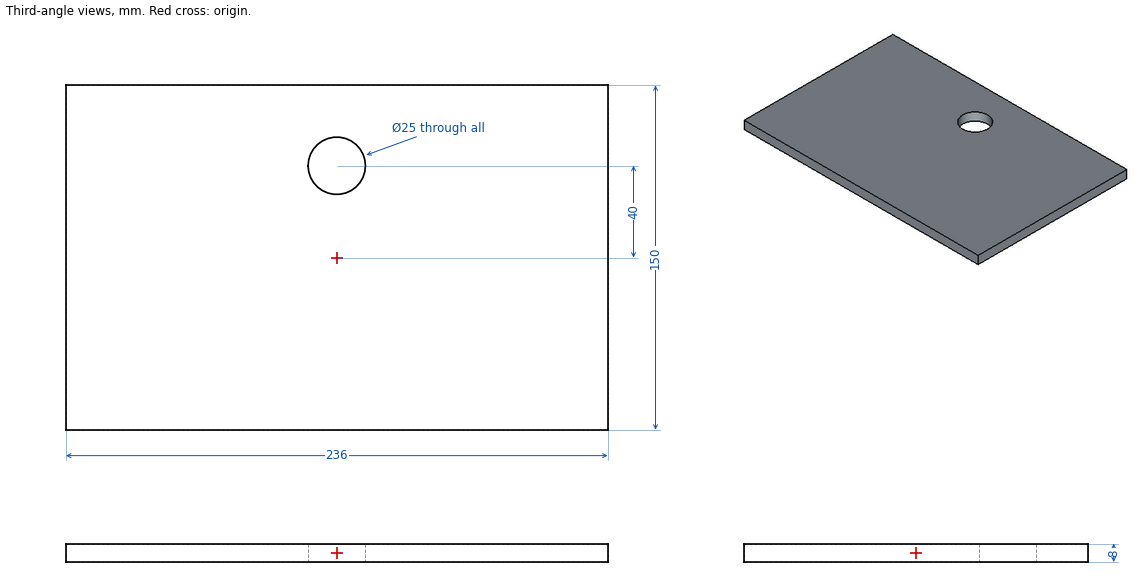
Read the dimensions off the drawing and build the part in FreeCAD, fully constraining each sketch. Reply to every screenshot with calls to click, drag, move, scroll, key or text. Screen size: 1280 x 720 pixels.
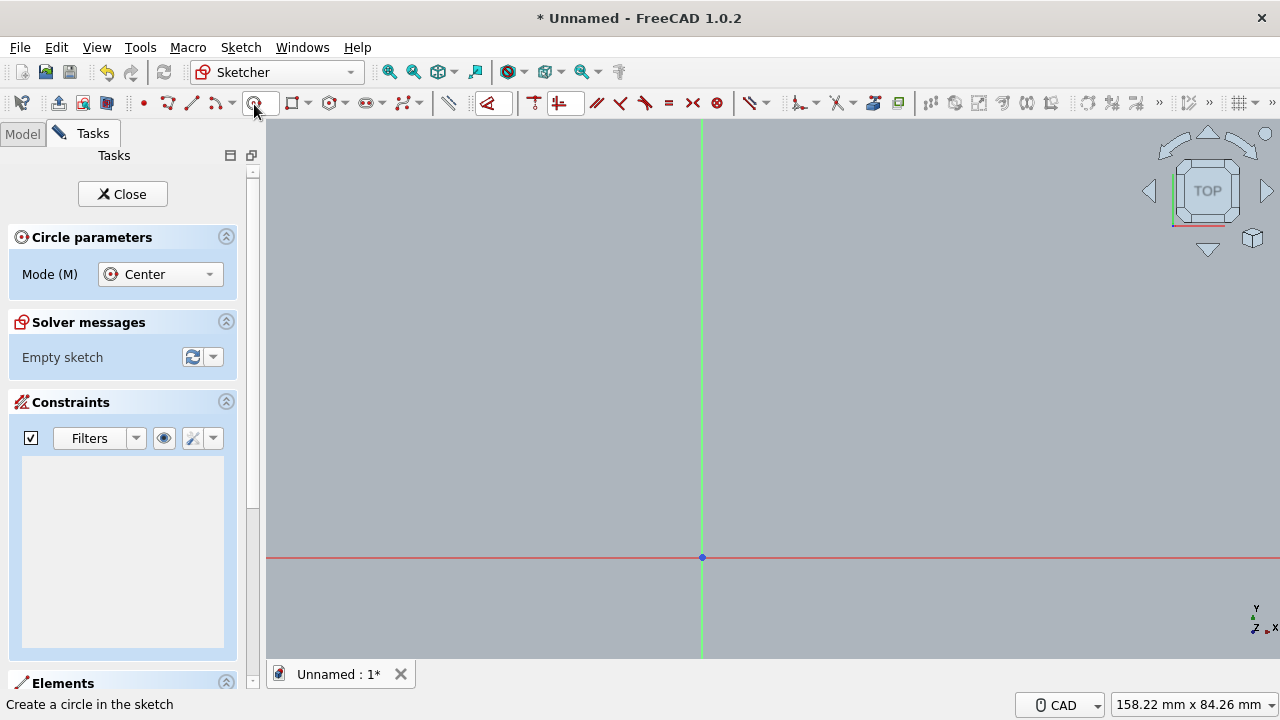
click(702, 301)
click(759, 245)
key(Escape)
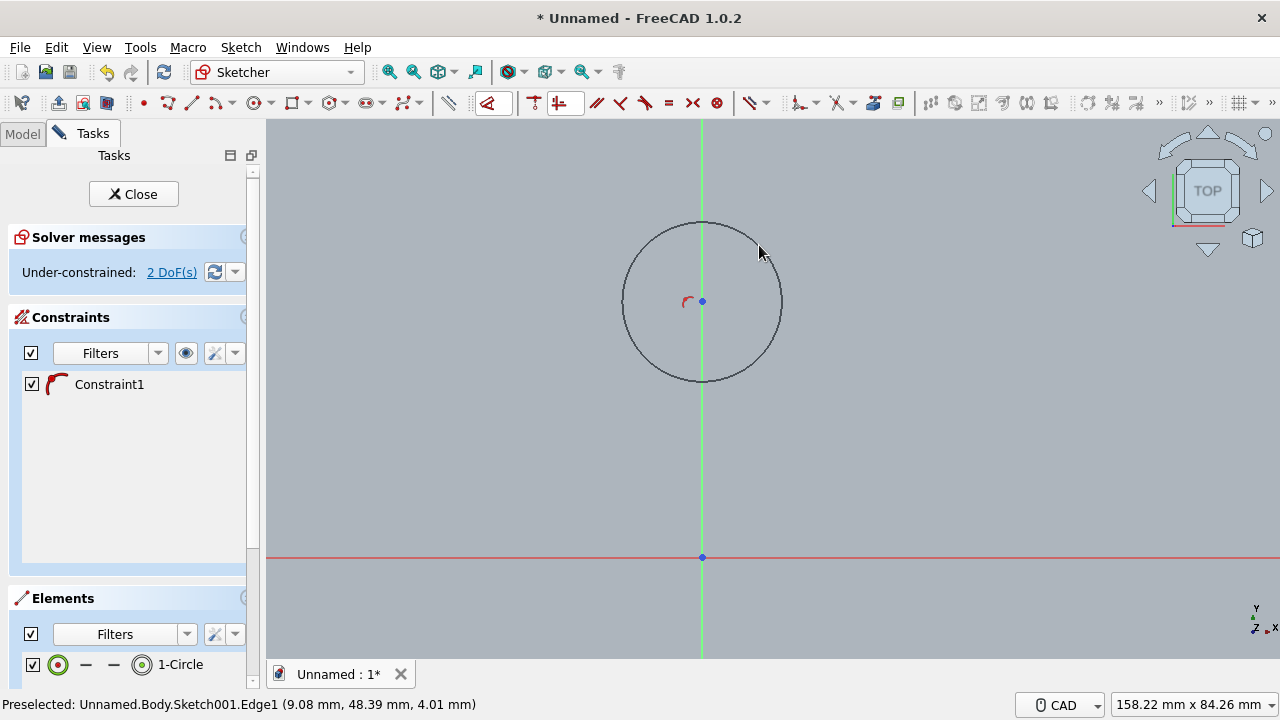
click(488, 104)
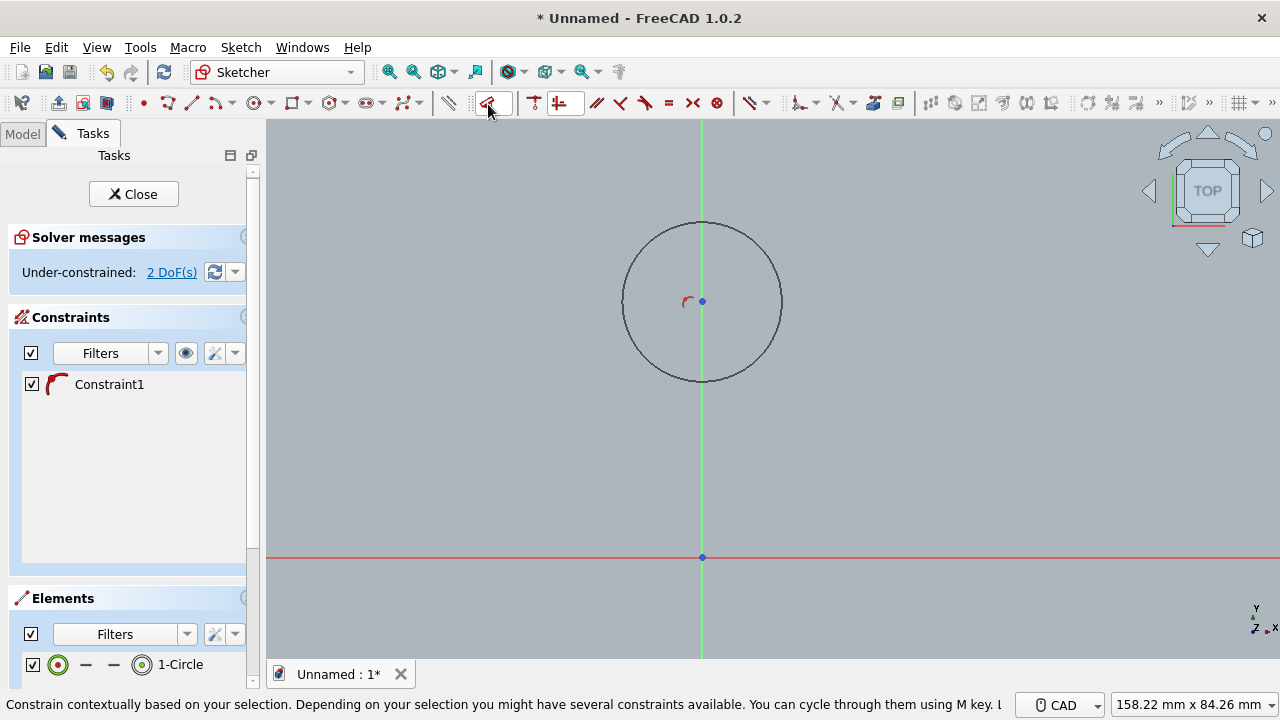
click(758, 245)
click(780, 222)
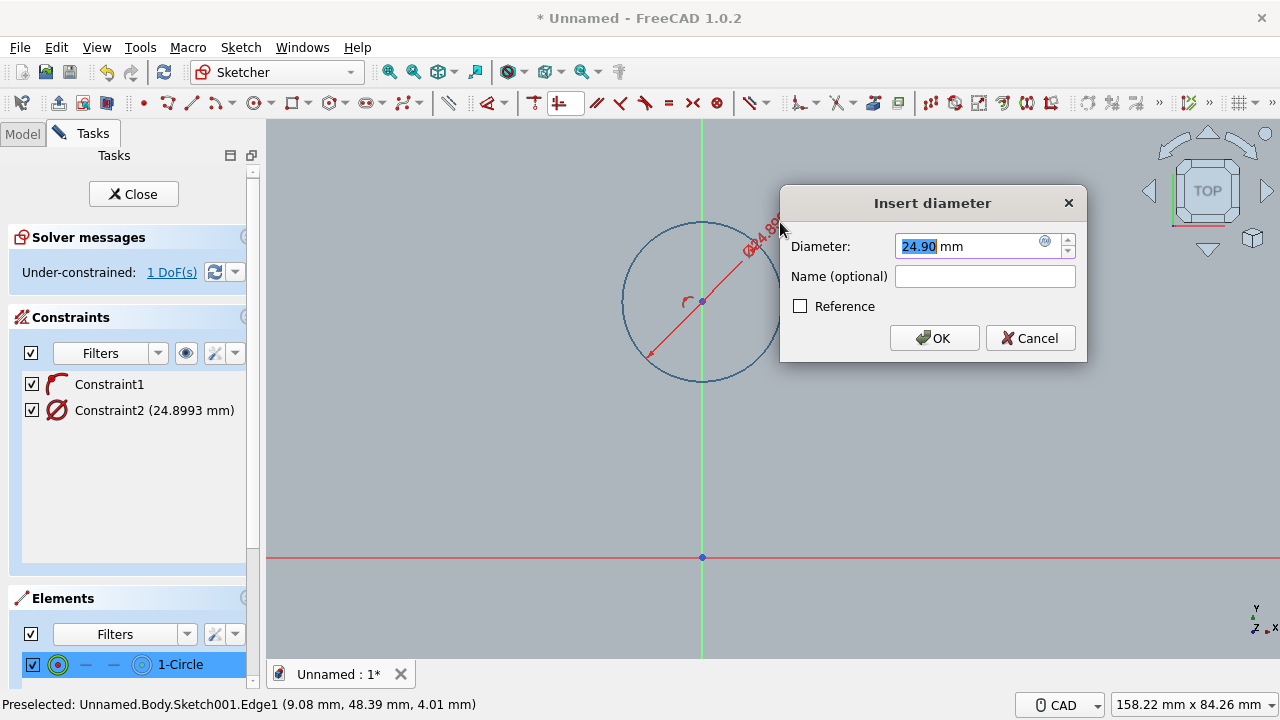
text(25)
key(Return)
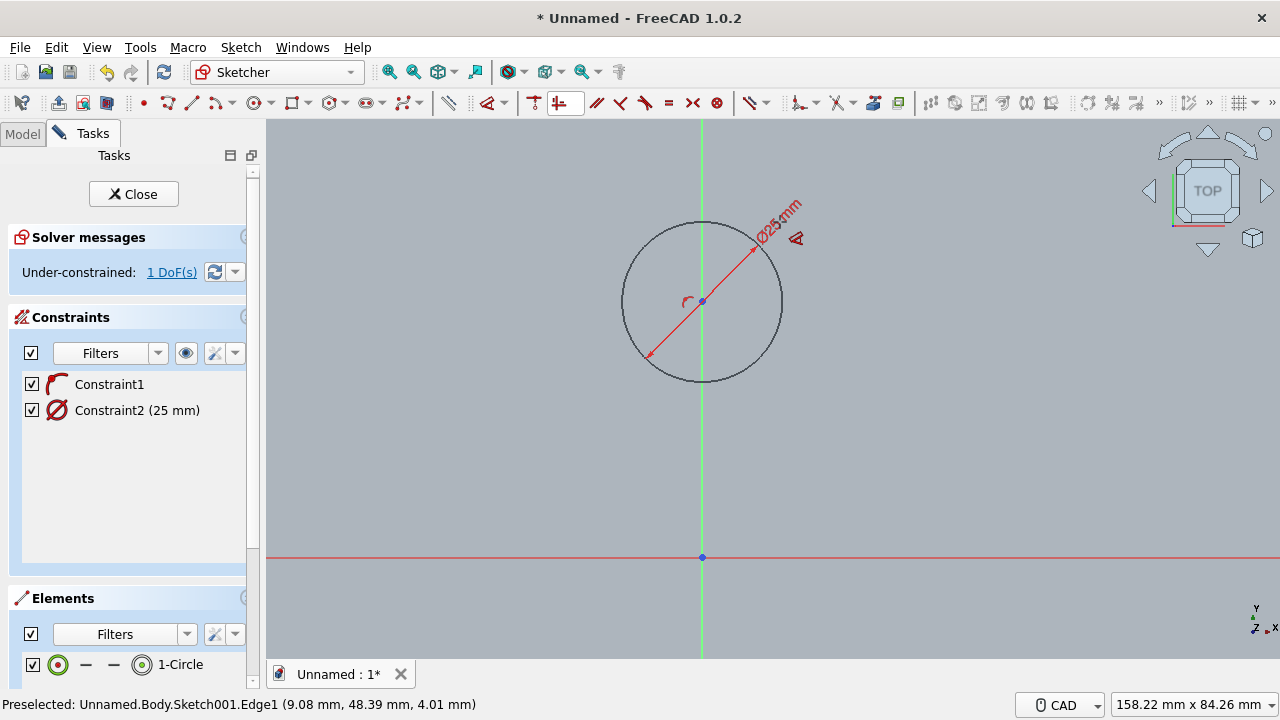
click(702, 302)
click(736, 430)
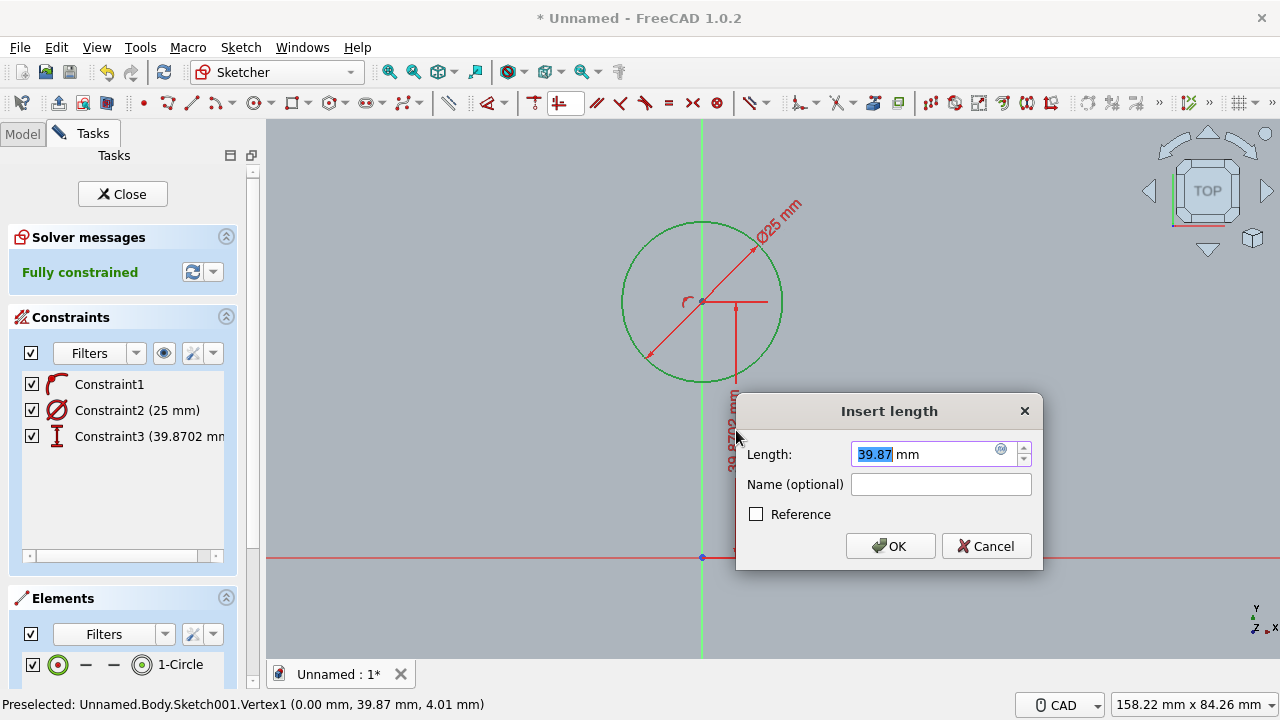
text(40)
key(Return)
key(Escape)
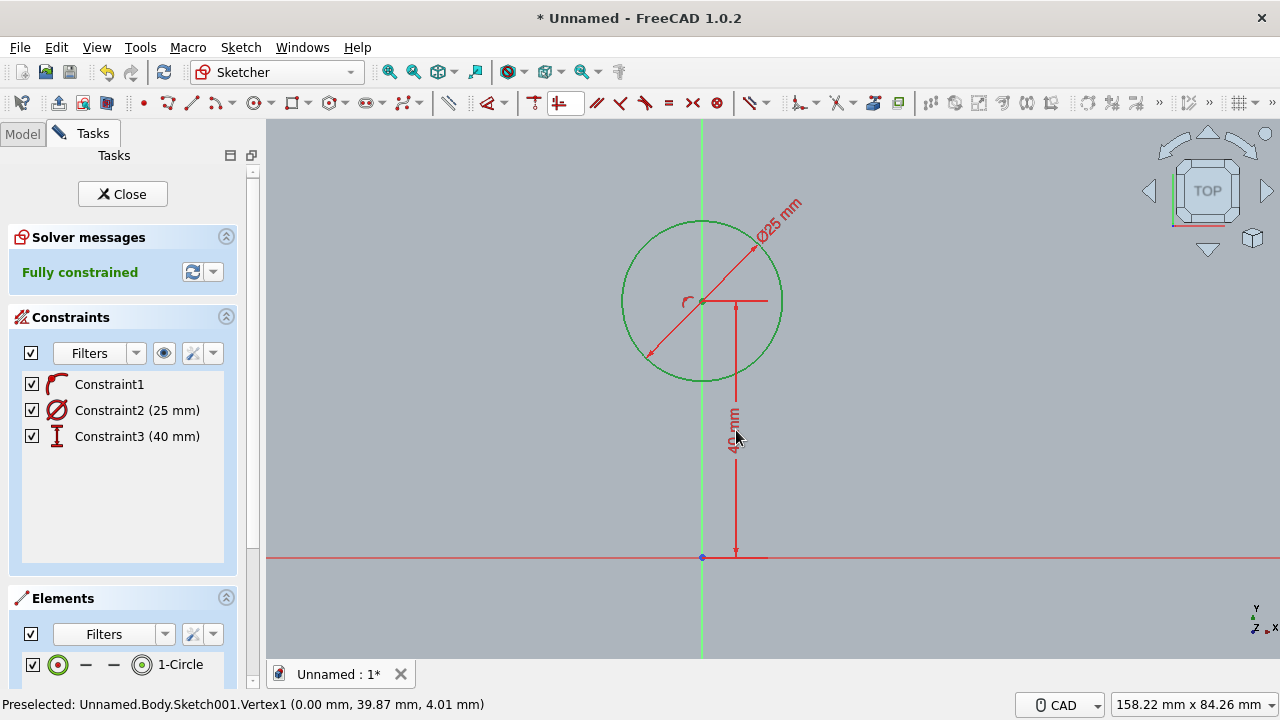
click(123, 194)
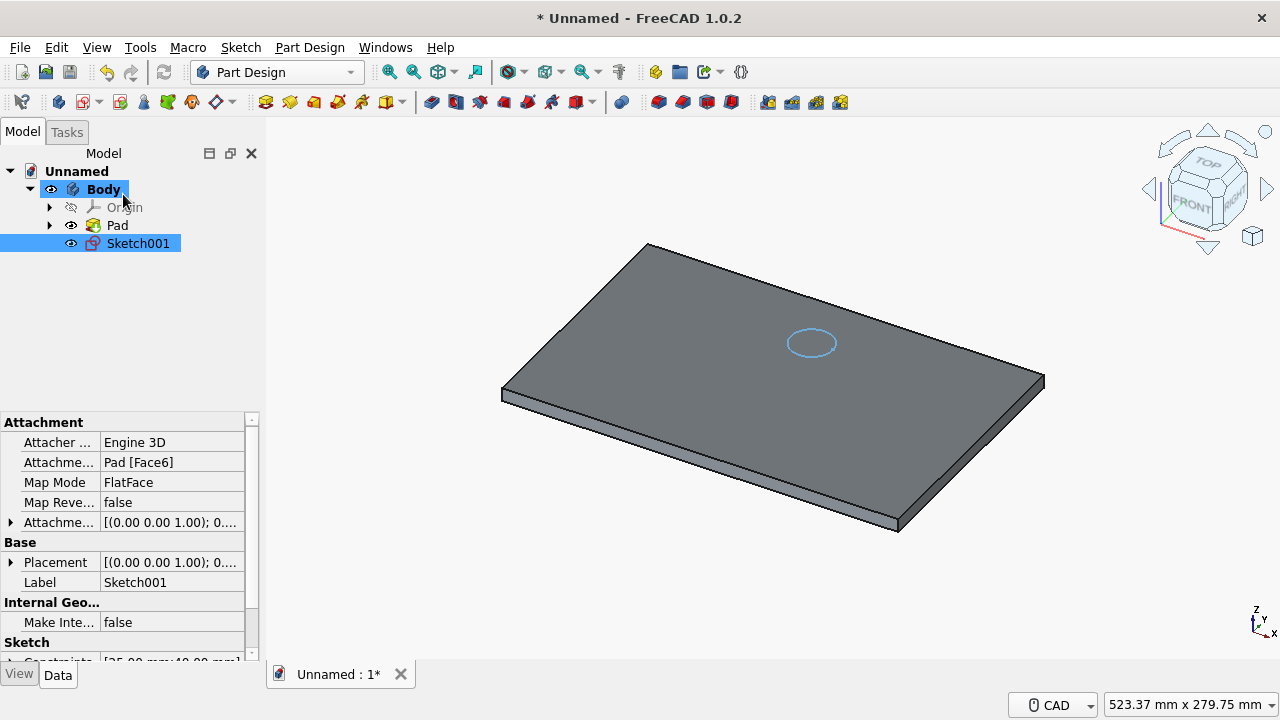
click(456, 102)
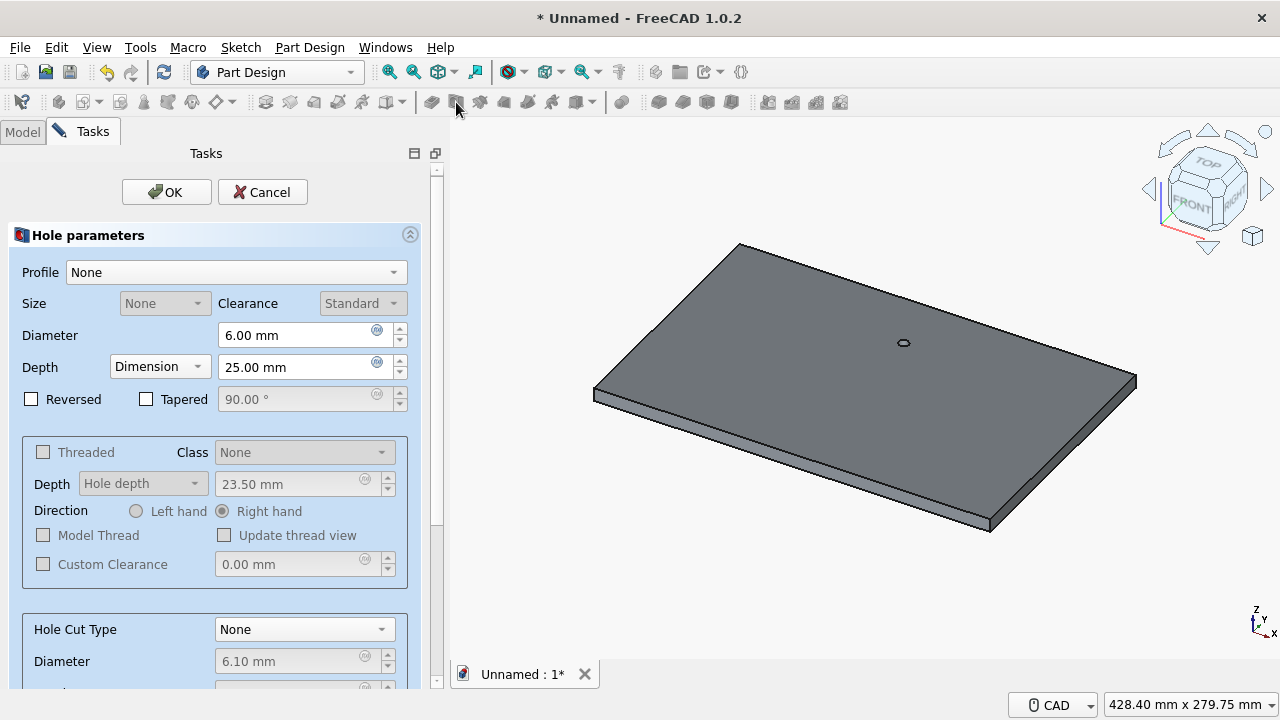
triple_click(305, 335)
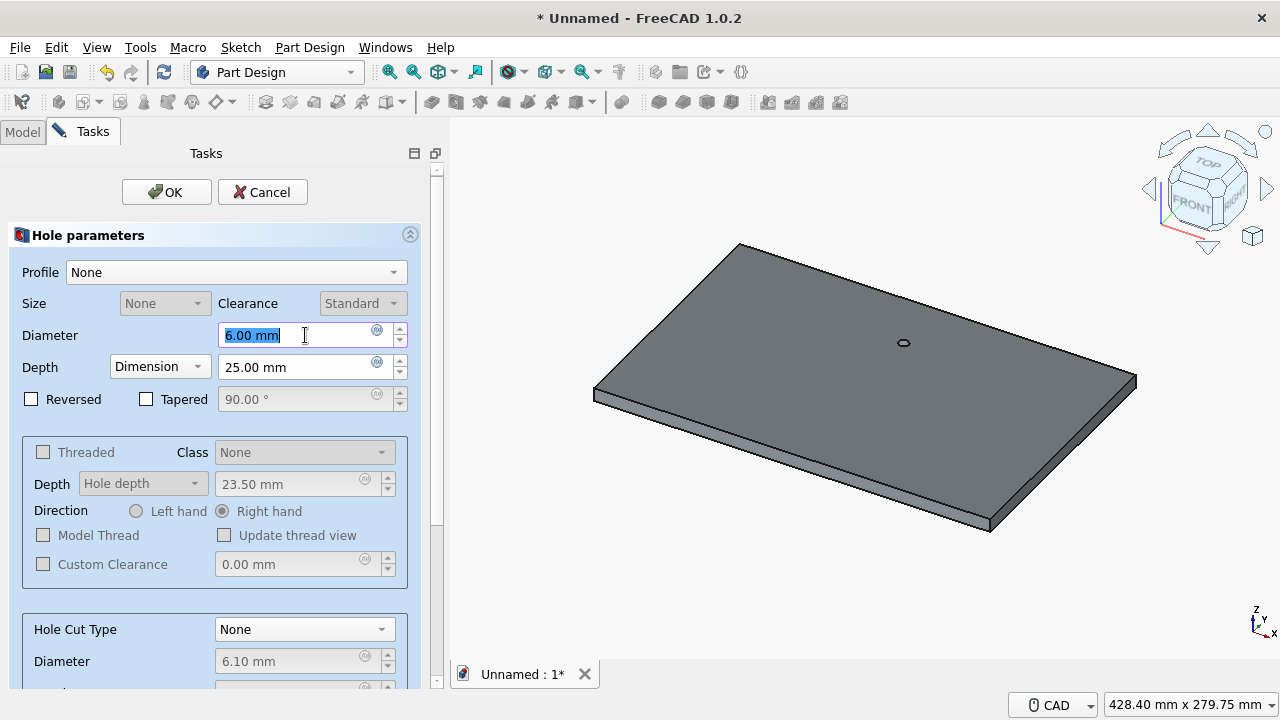
text(25)
key(Tab)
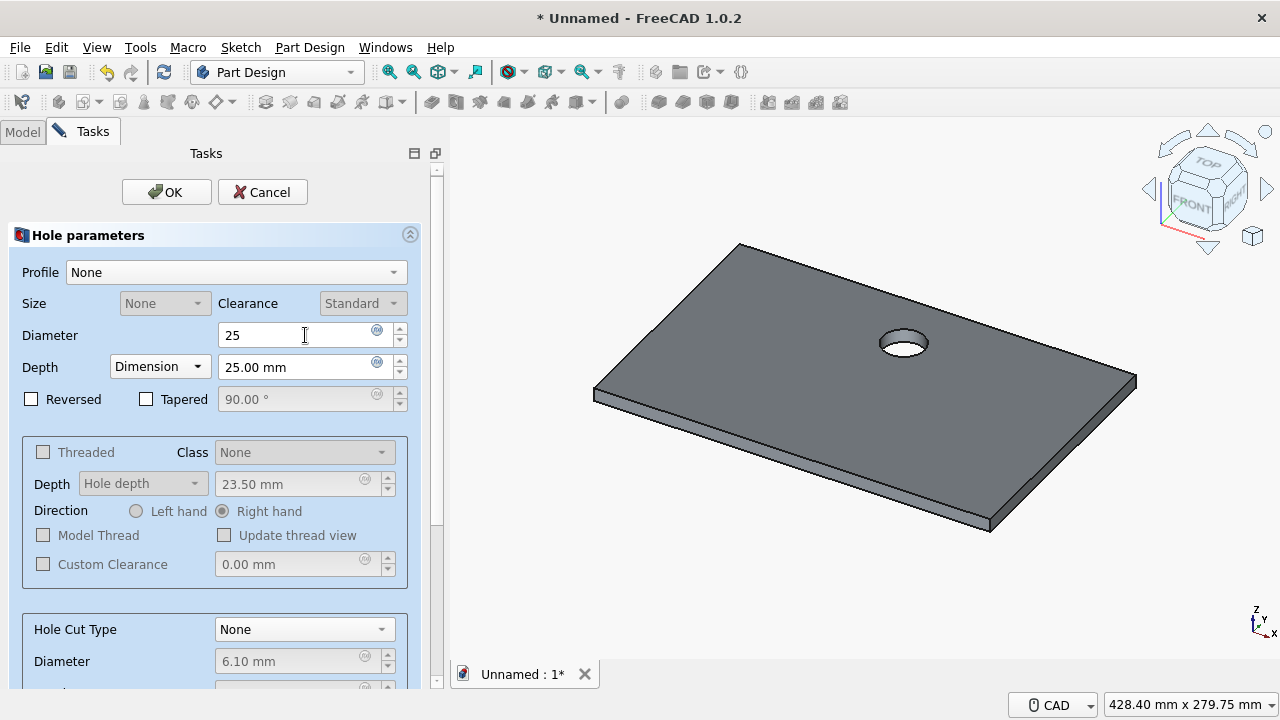
click(161, 366)